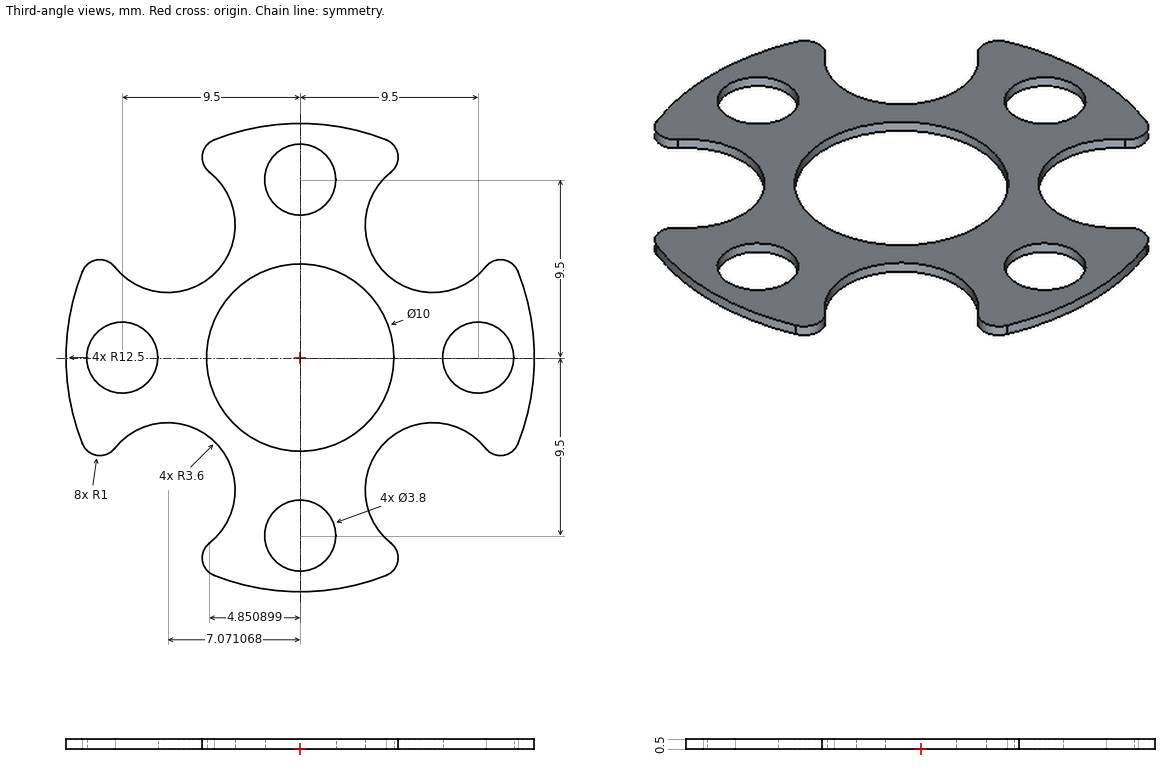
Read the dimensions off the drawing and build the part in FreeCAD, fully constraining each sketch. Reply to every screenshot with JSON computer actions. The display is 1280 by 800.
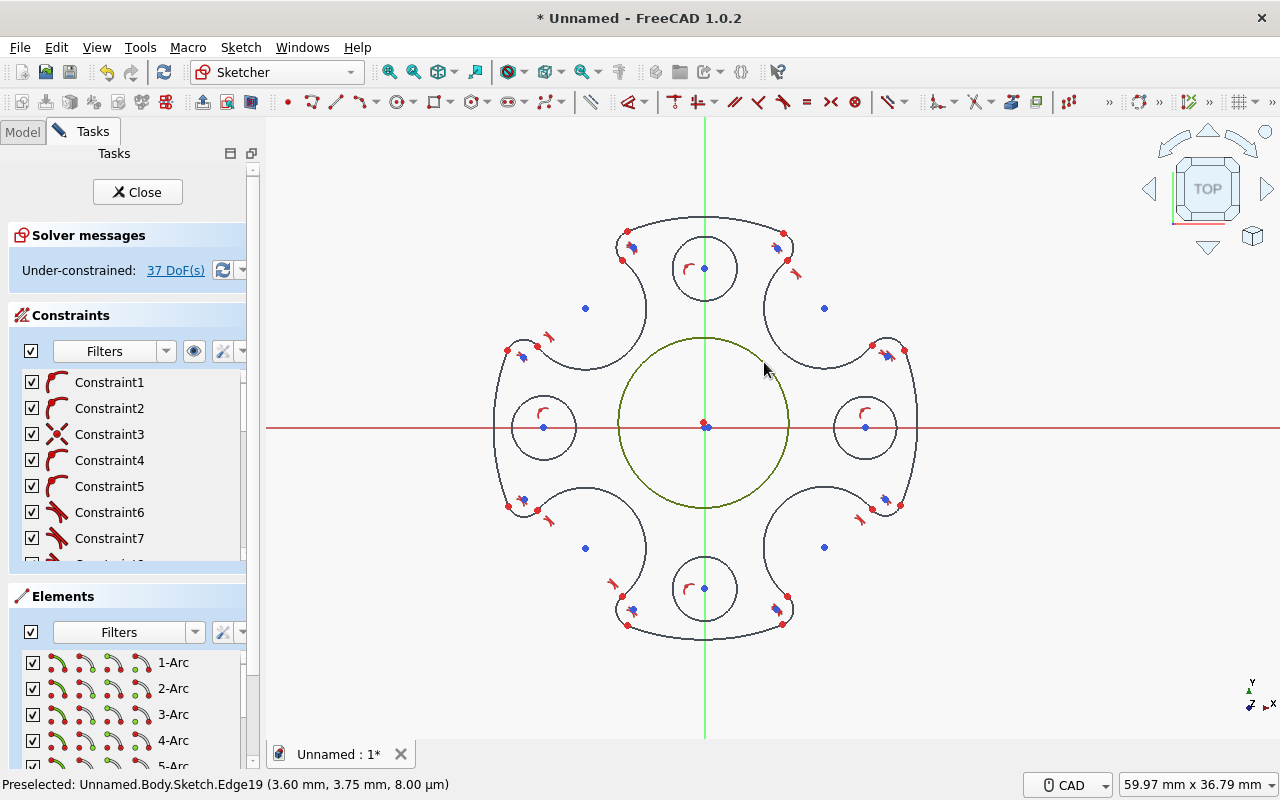
{"action": "left_click", "coordinate": [496, 397]}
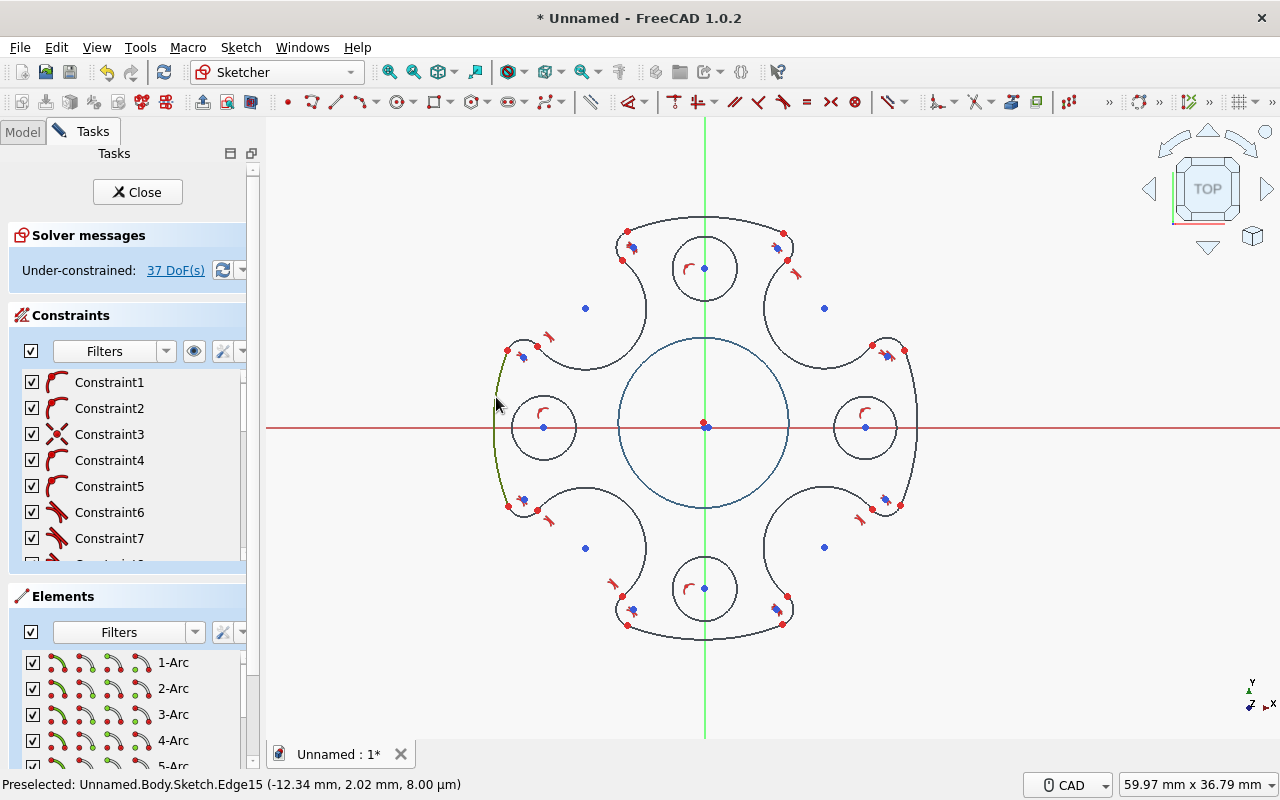
{"action": "key", "text": "c"}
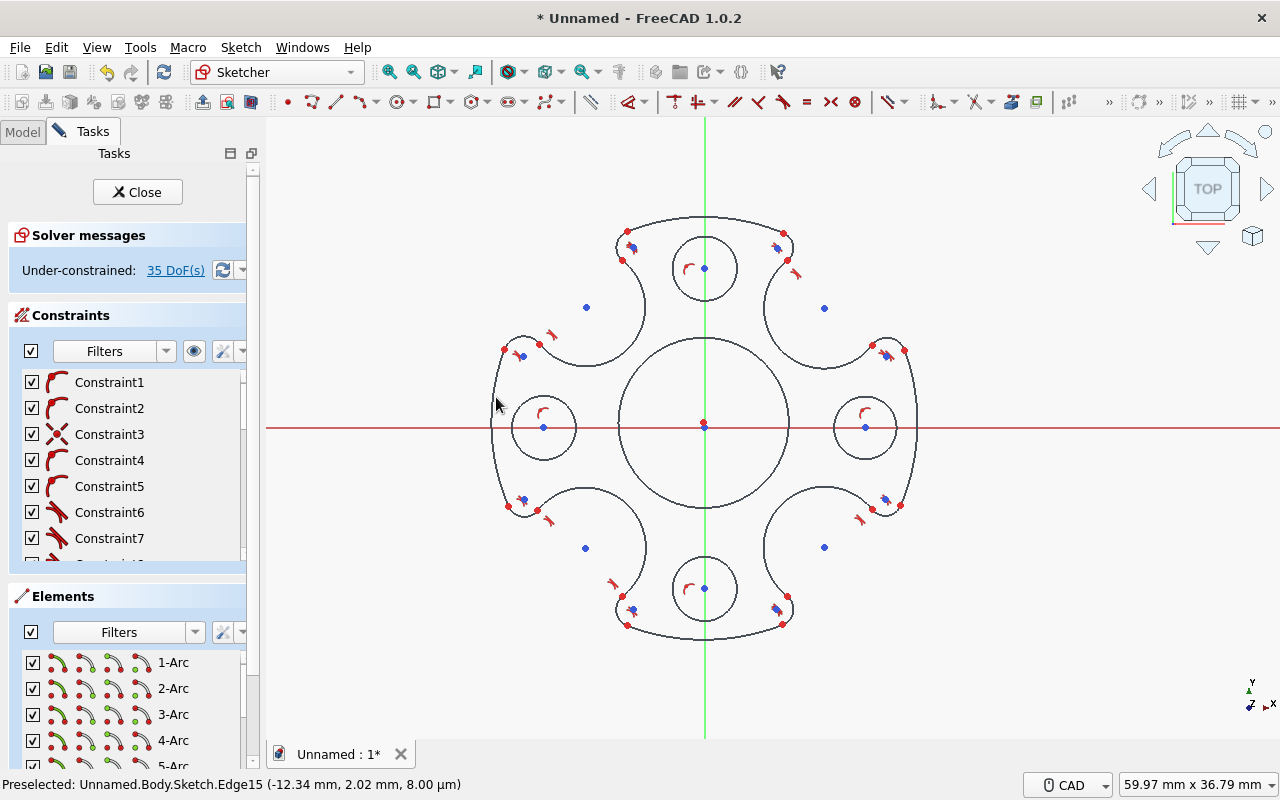
{"action": "scroll", "coordinate": [704, 425], "scroll_direction": "up", "scroll_amount": 5}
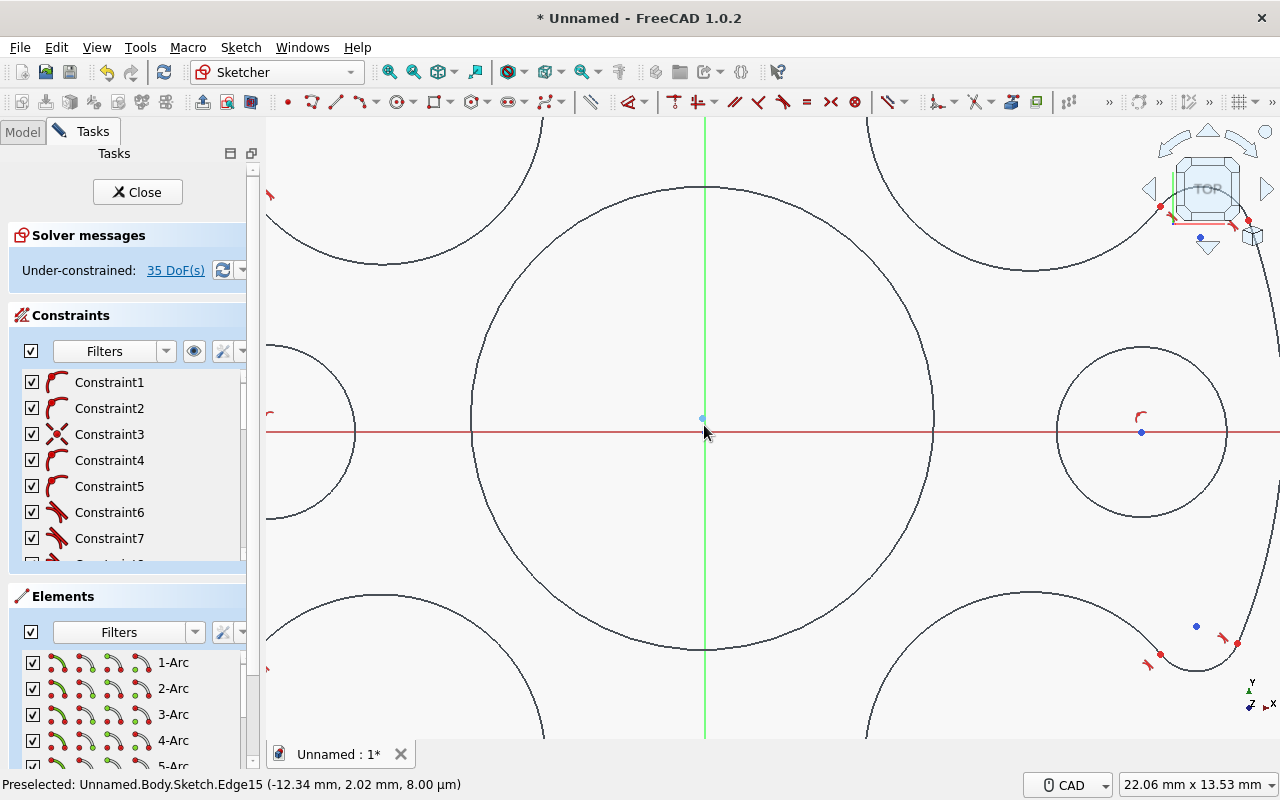
{"action": "left_click_drag", "start_coordinate": [692, 408], "coordinate": [715, 442]}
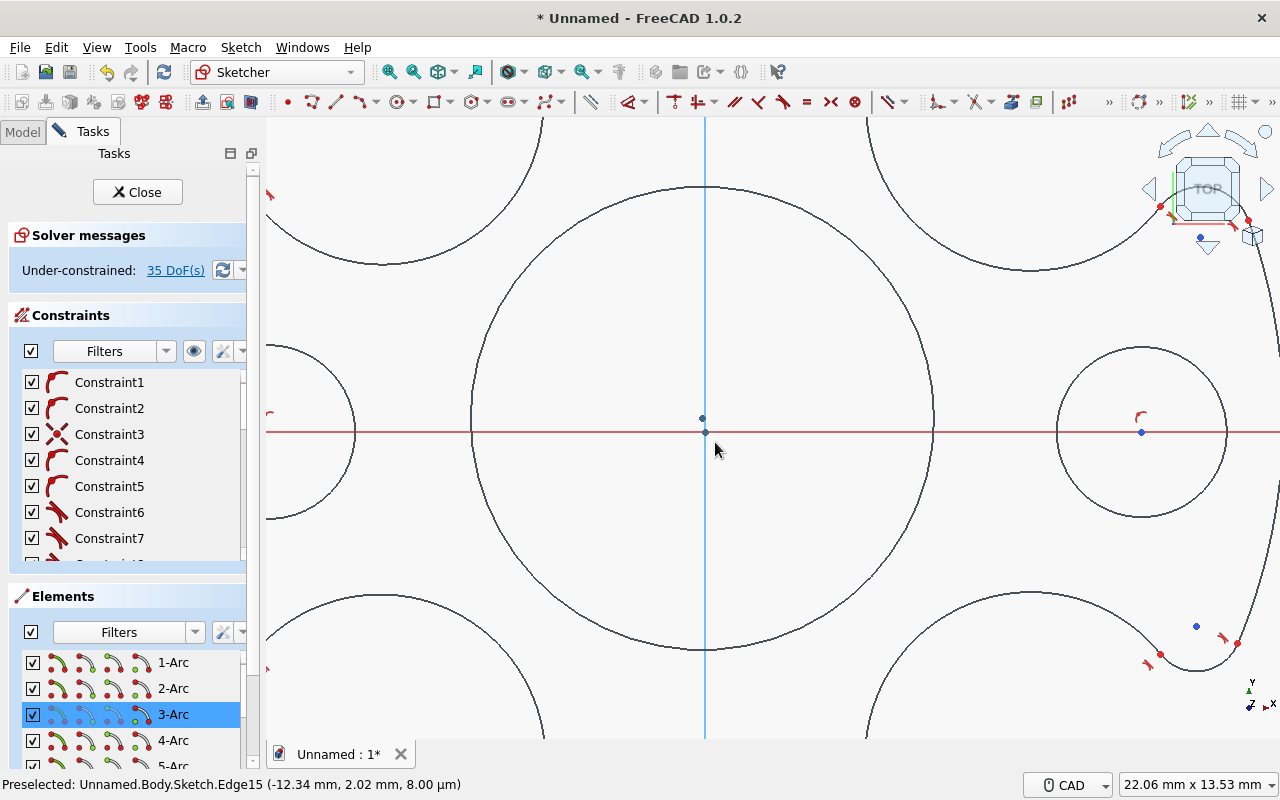
{"action": "key", "text": "c"}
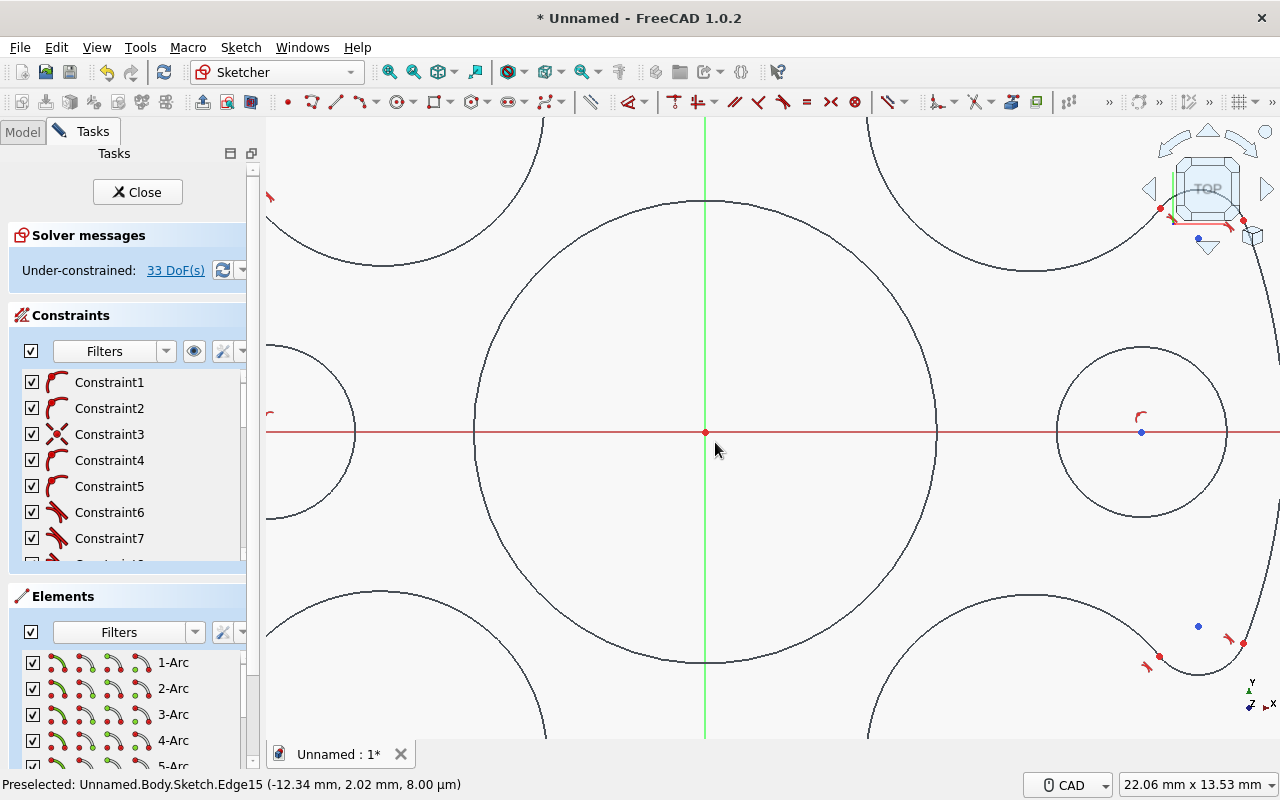
{"action": "scroll", "coordinate": [704, 426], "scroll_direction": "down", "scroll_amount": 5}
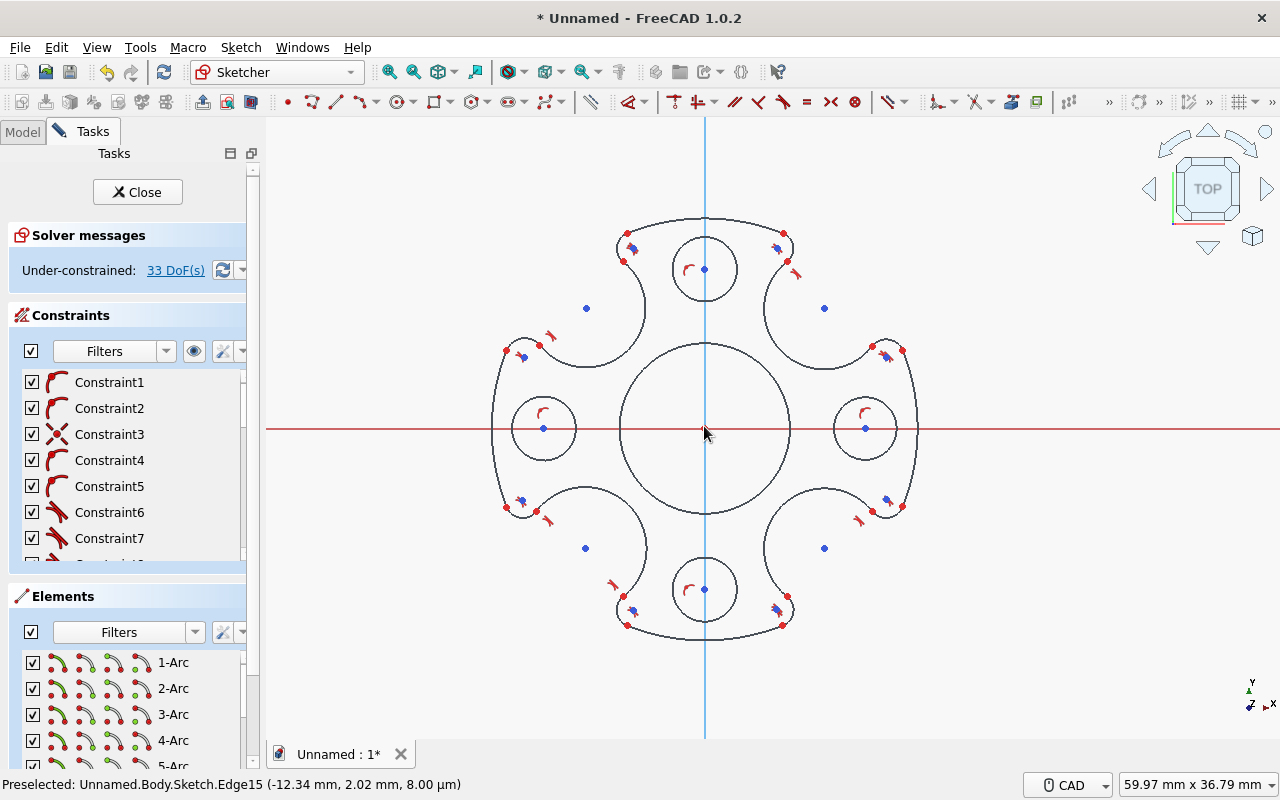
{"action": "scroll", "coordinate": [617, 605], "scroll_direction": "up", "scroll_amount": 2}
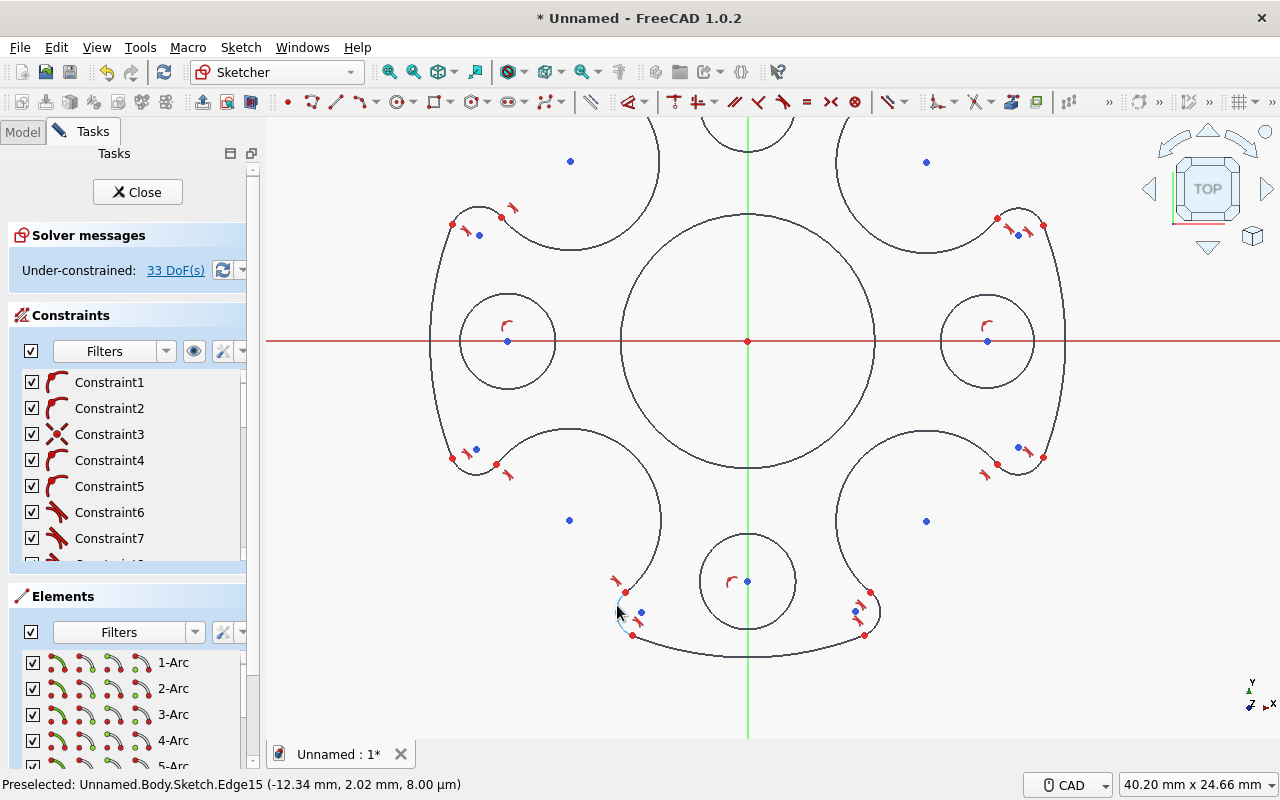
{"action": "left_click", "coordinate": [617, 605]}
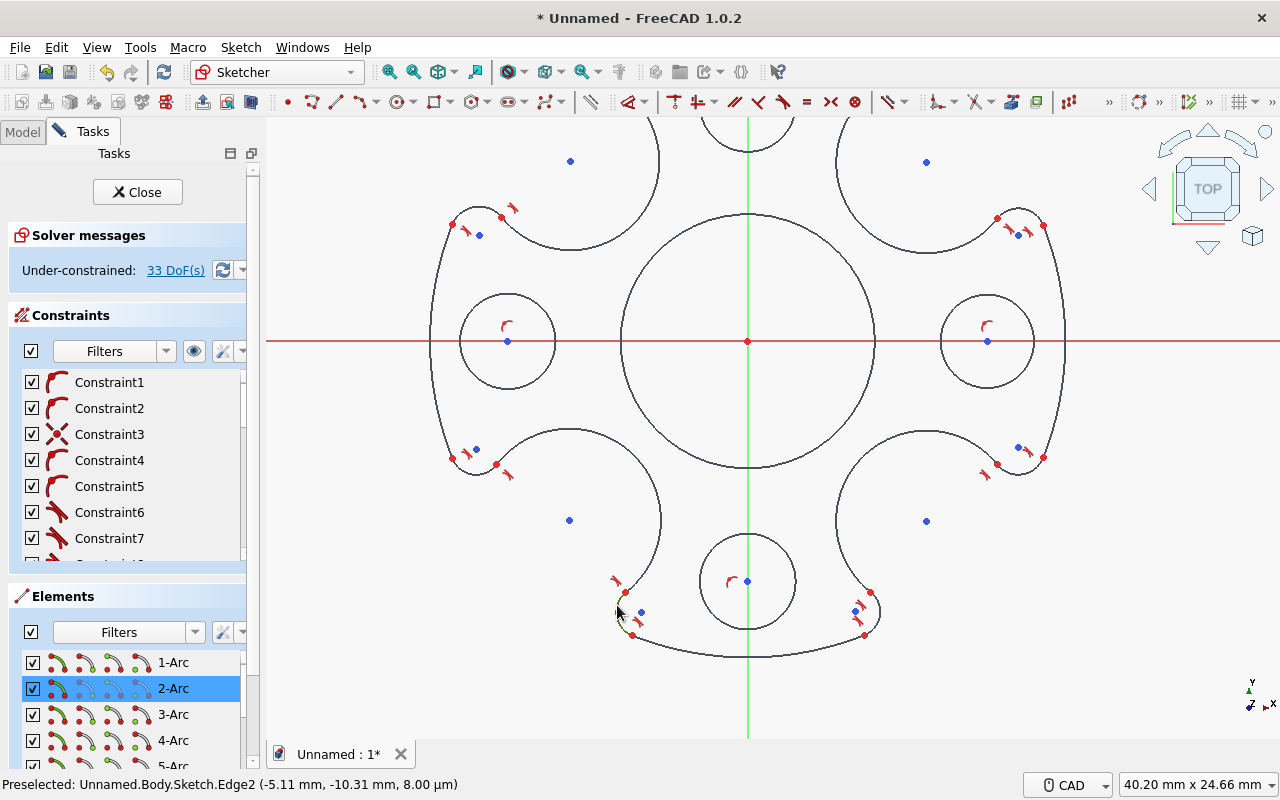
{"action": "left_click", "coordinate": [876, 625]}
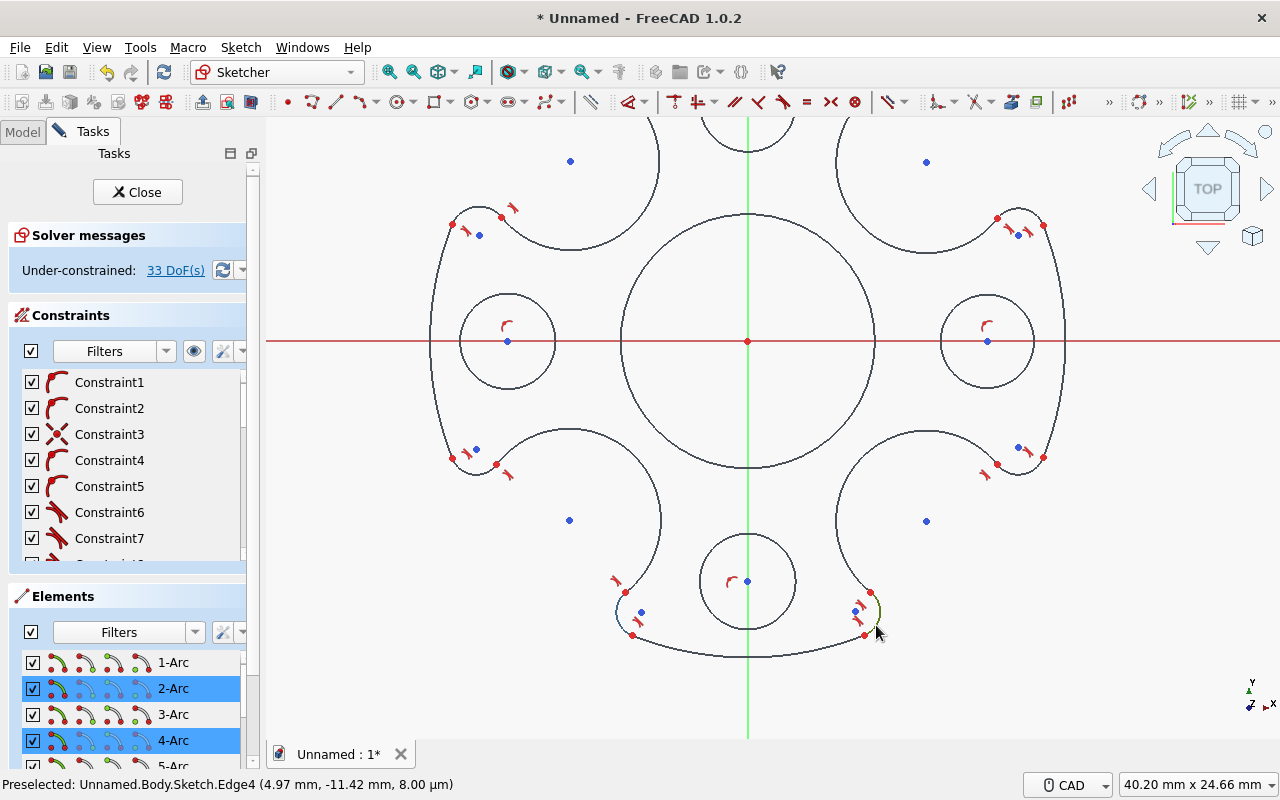
{"action": "left_click", "coordinate": [1011, 474]}